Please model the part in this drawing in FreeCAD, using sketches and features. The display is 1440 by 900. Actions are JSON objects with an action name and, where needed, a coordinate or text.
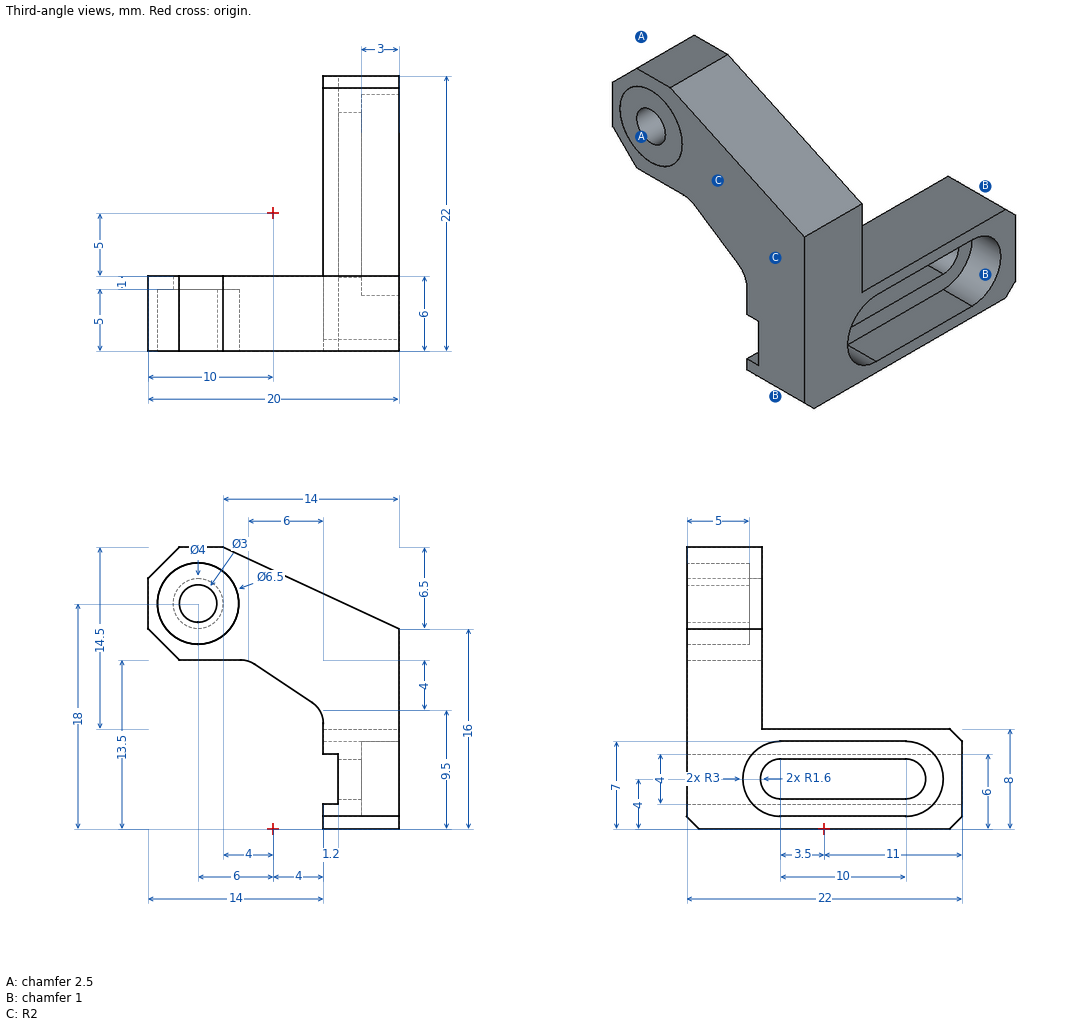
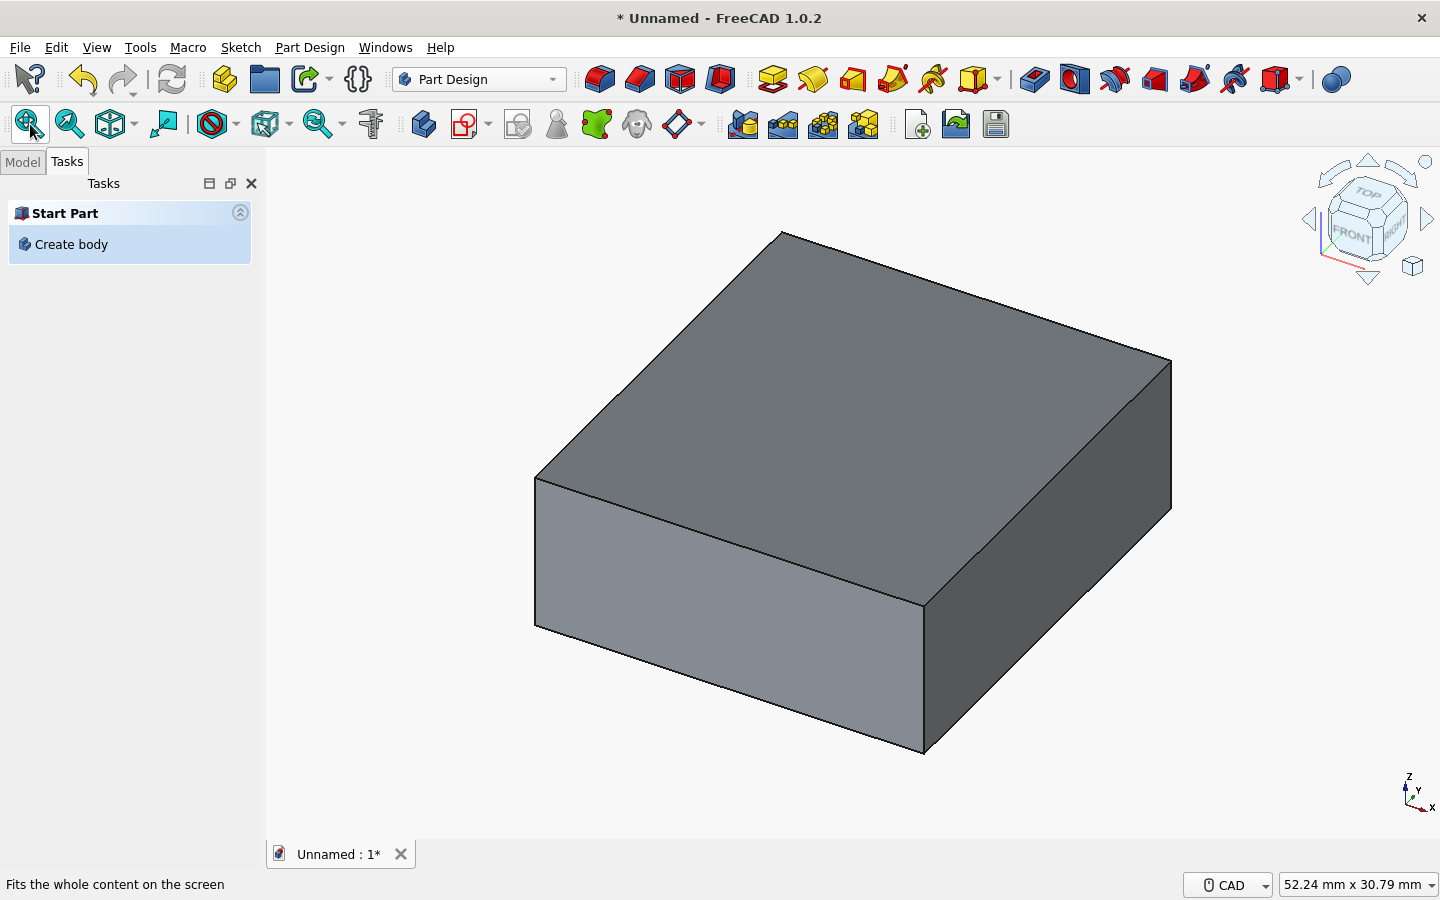
{"action": "left_click", "coordinate": [853, 418]}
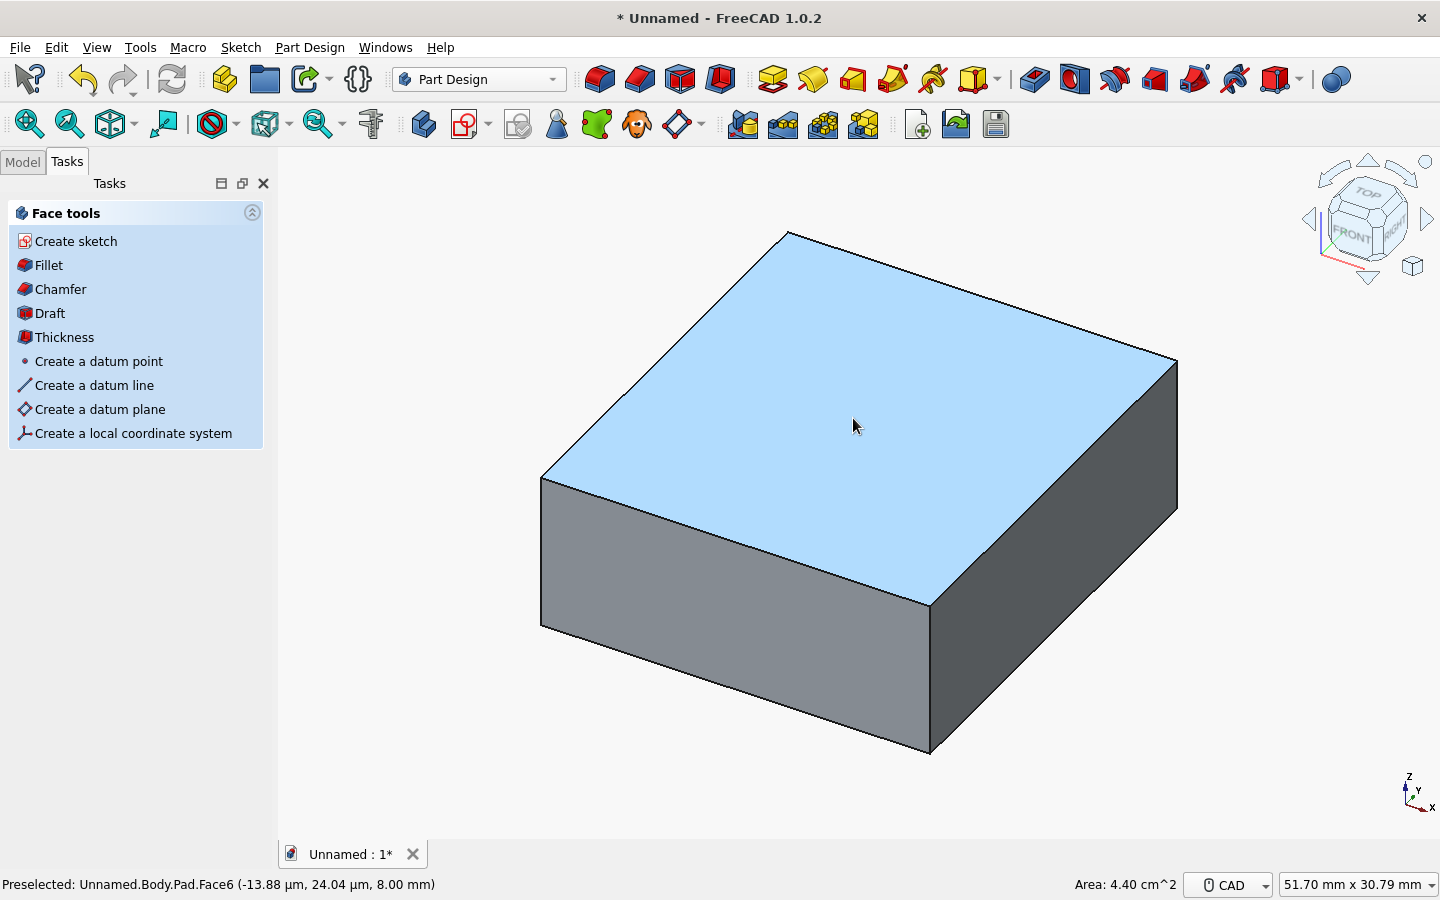
{"action": "left_click", "coordinate": [464, 124]}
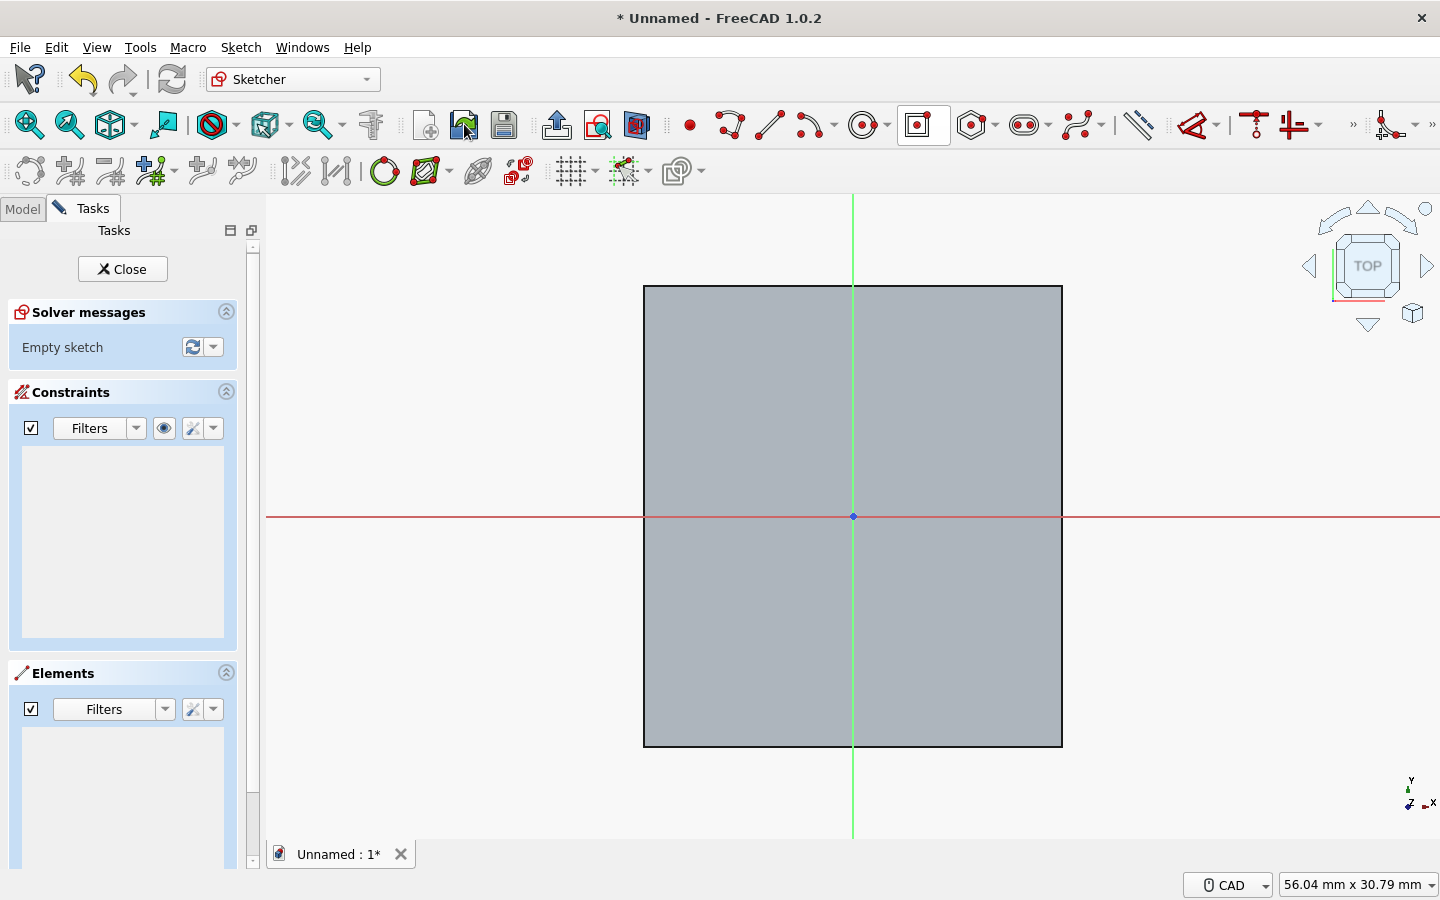
{"action": "scroll", "coordinate": [936, 772], "scroll_direction": "up", "scroll_amount": 3}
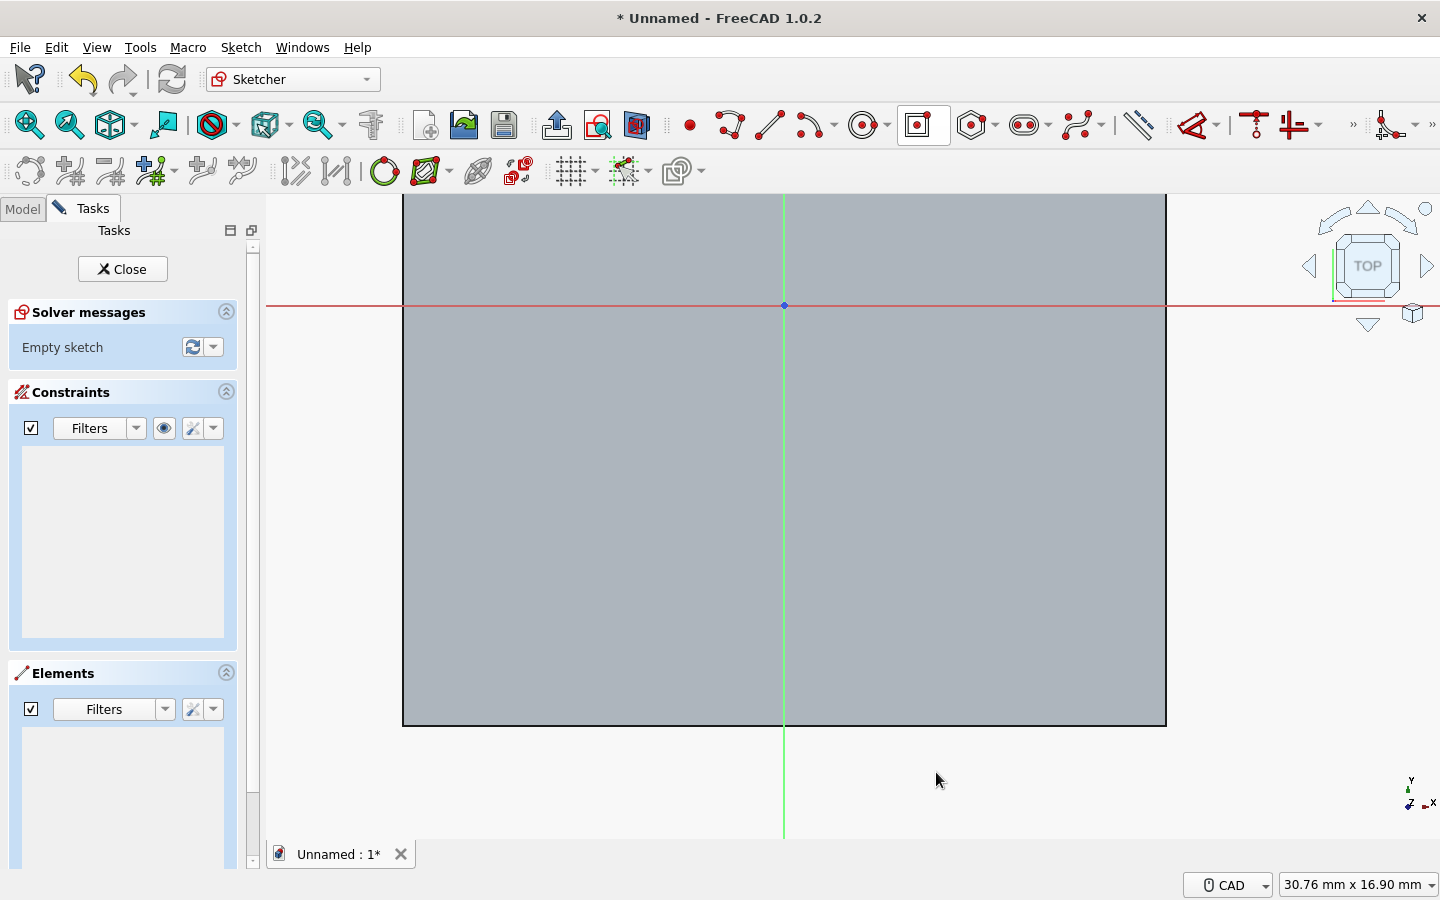
{"action": "key", "text": "g r"}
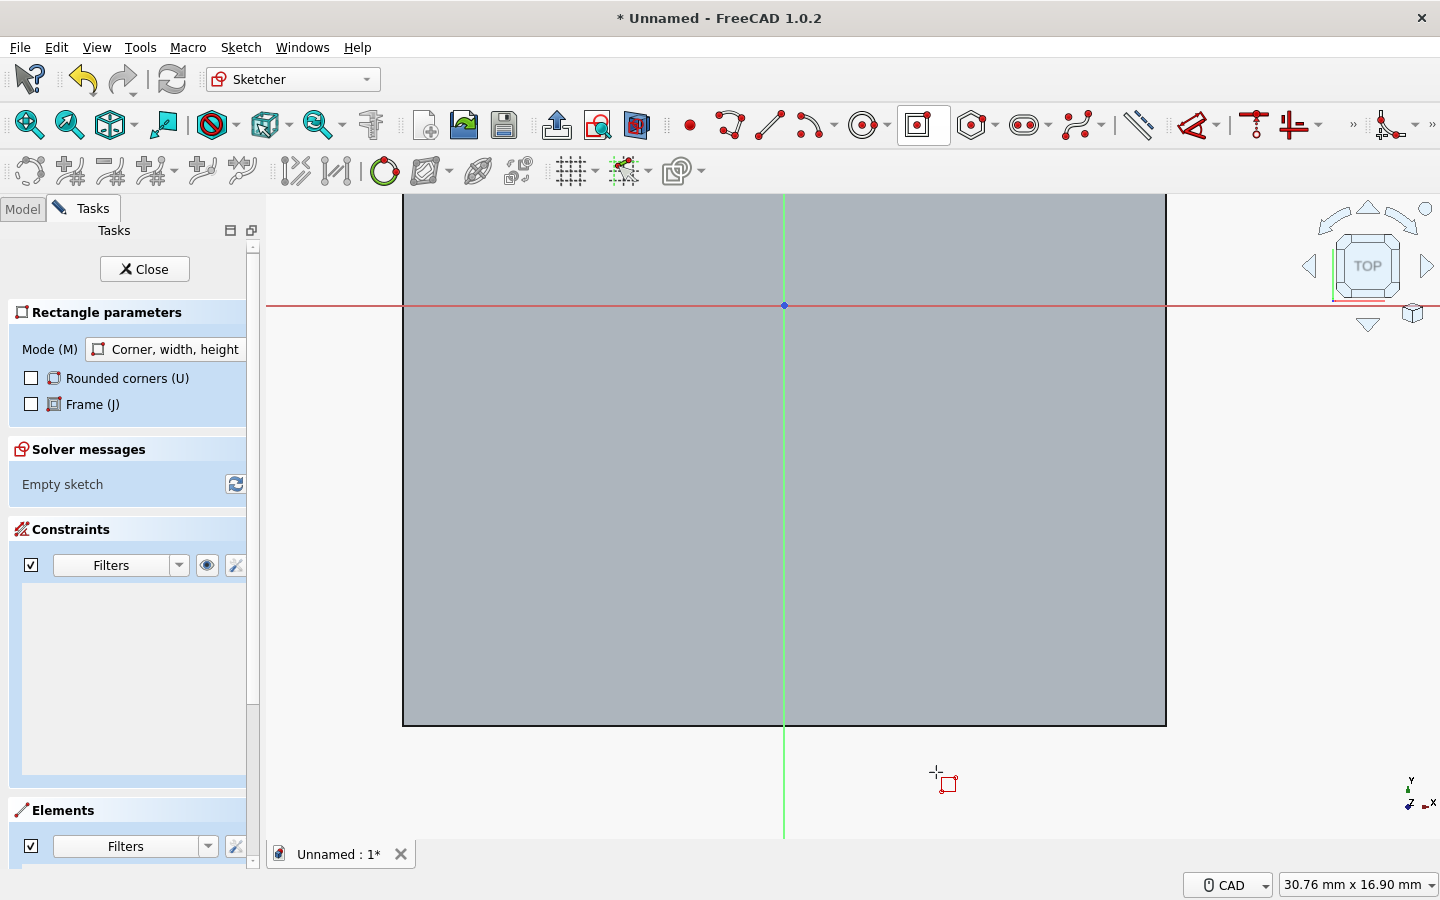
{"action": "left_click", "coordinate": [403, 497]}
{"action": "mouse_move", "coordinate": [1166, 726]}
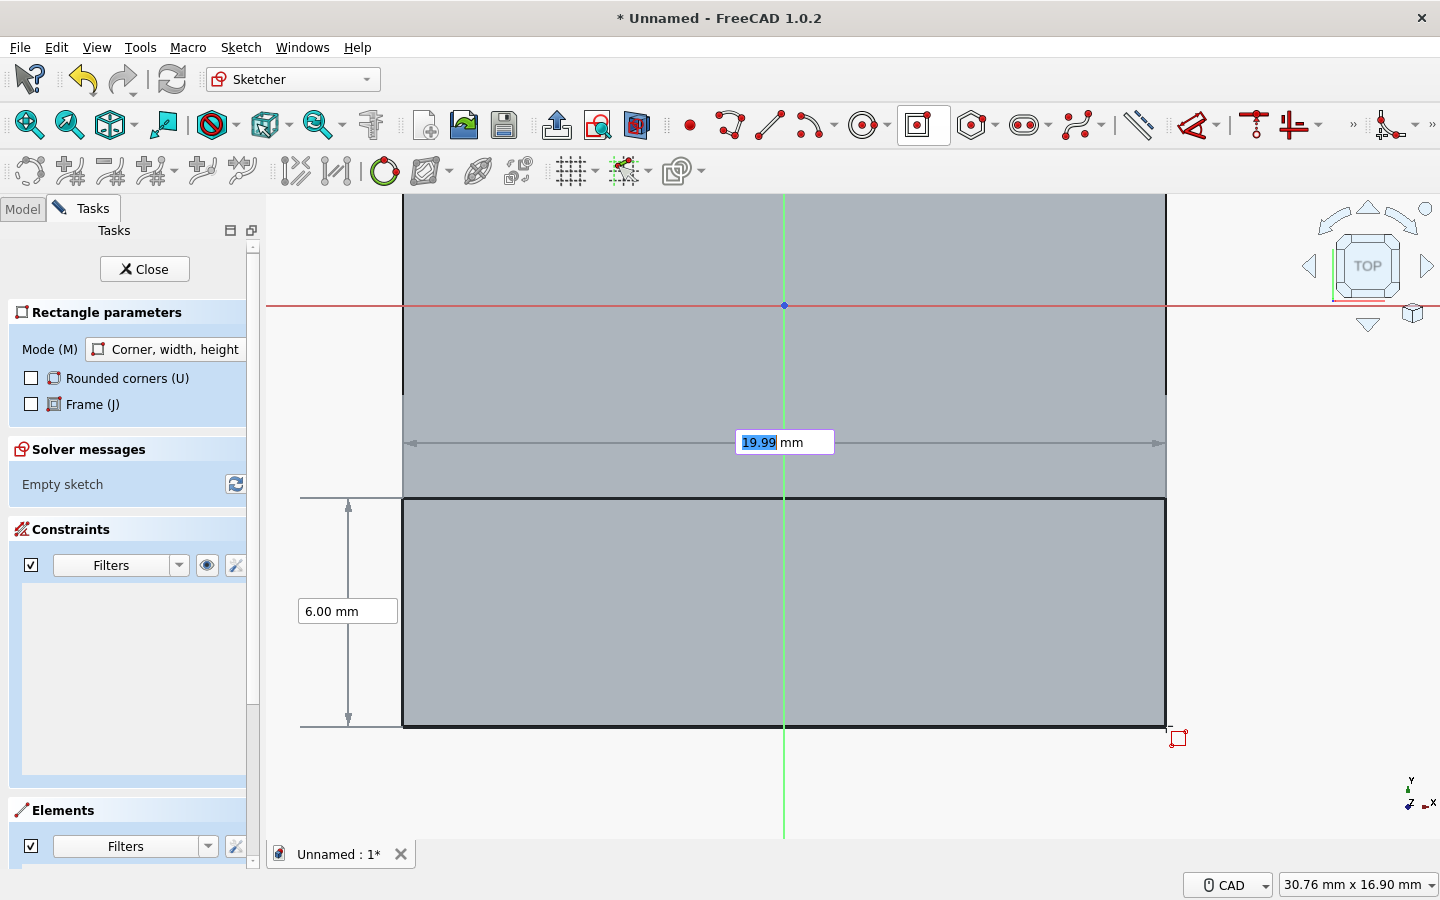
{"action": "type", "text": "20"}
{"action": "key", "text": "Tab"}
{"action": "type", "text": "6"}
{"action": "key", "text": "Return"}
{"action": "key", "text": "Escape"}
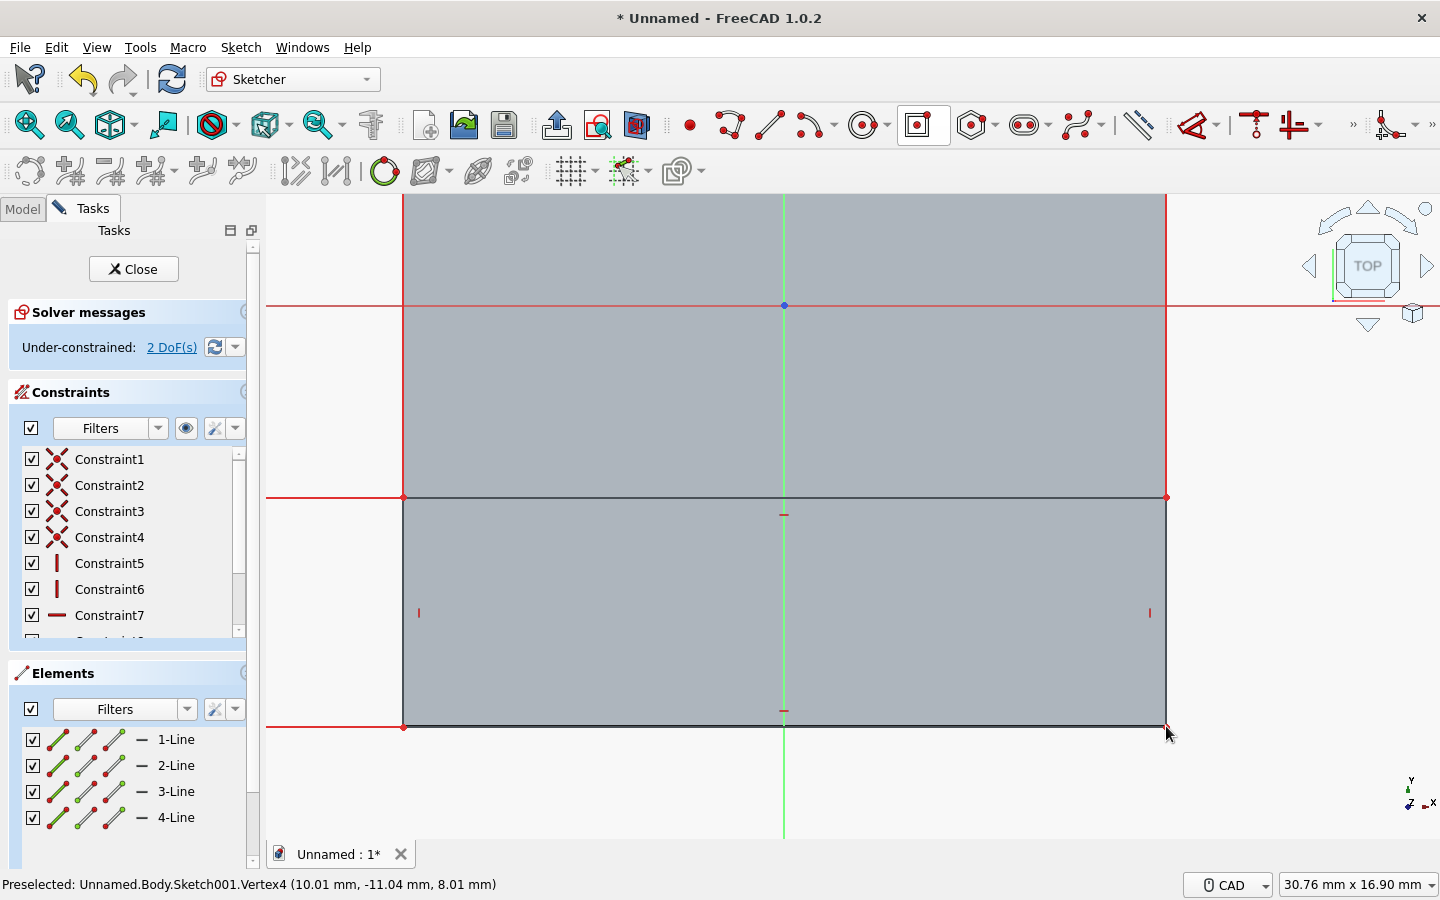
{"action": "left_click", "coordinate": [1192, 126]}